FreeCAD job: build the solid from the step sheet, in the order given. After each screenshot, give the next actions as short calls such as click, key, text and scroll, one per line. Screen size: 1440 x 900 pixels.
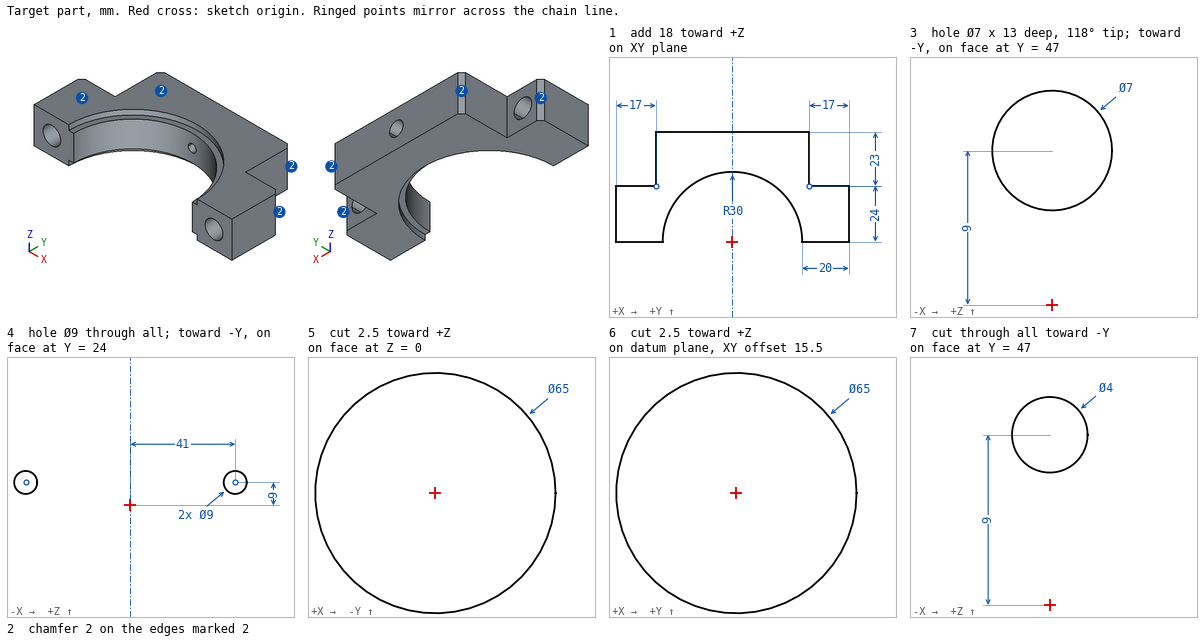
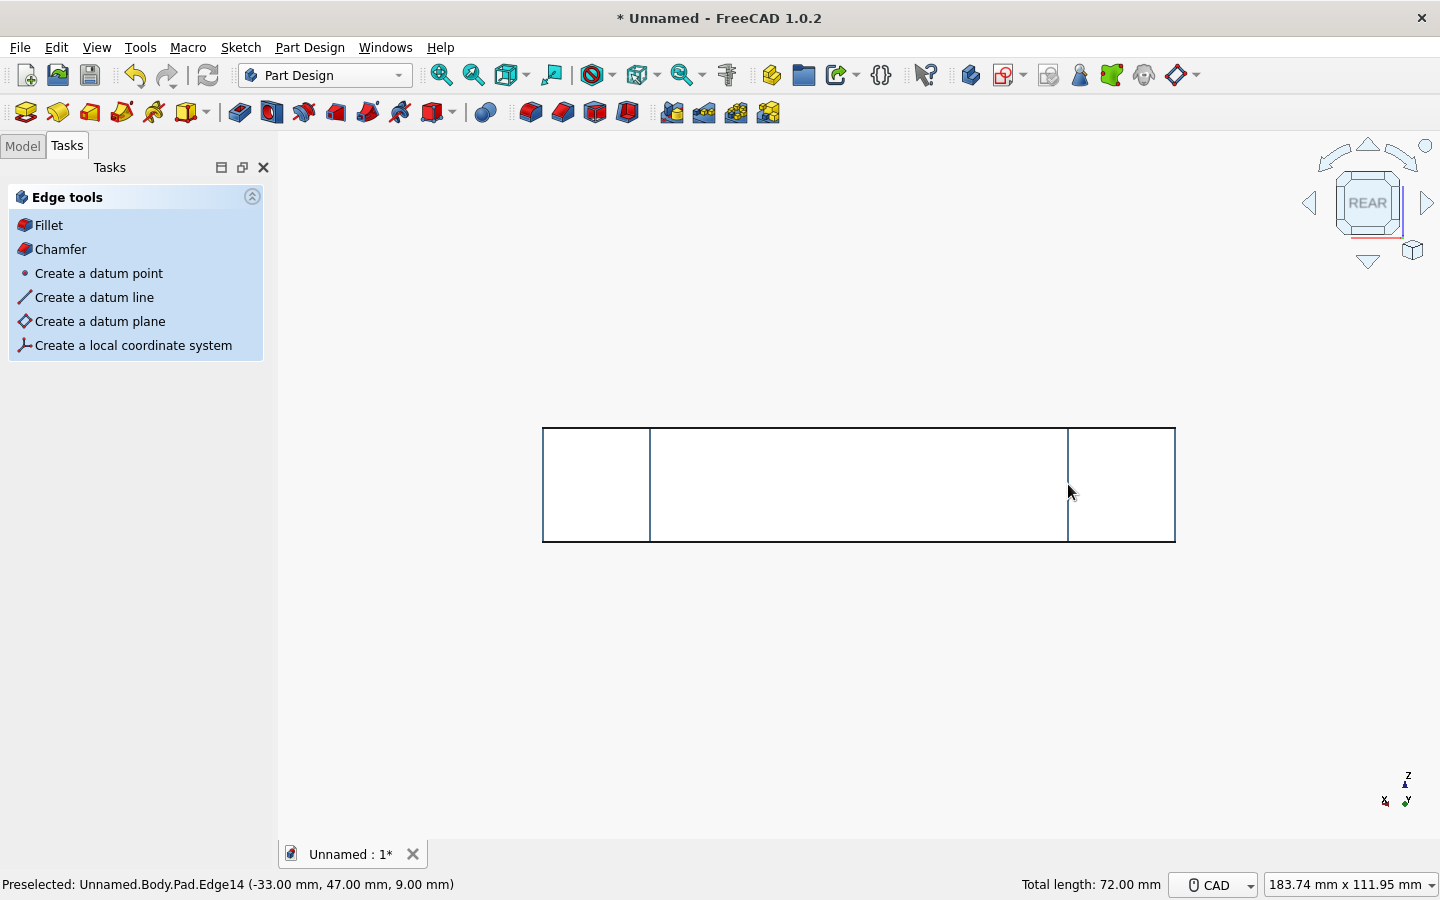
click(564, 112)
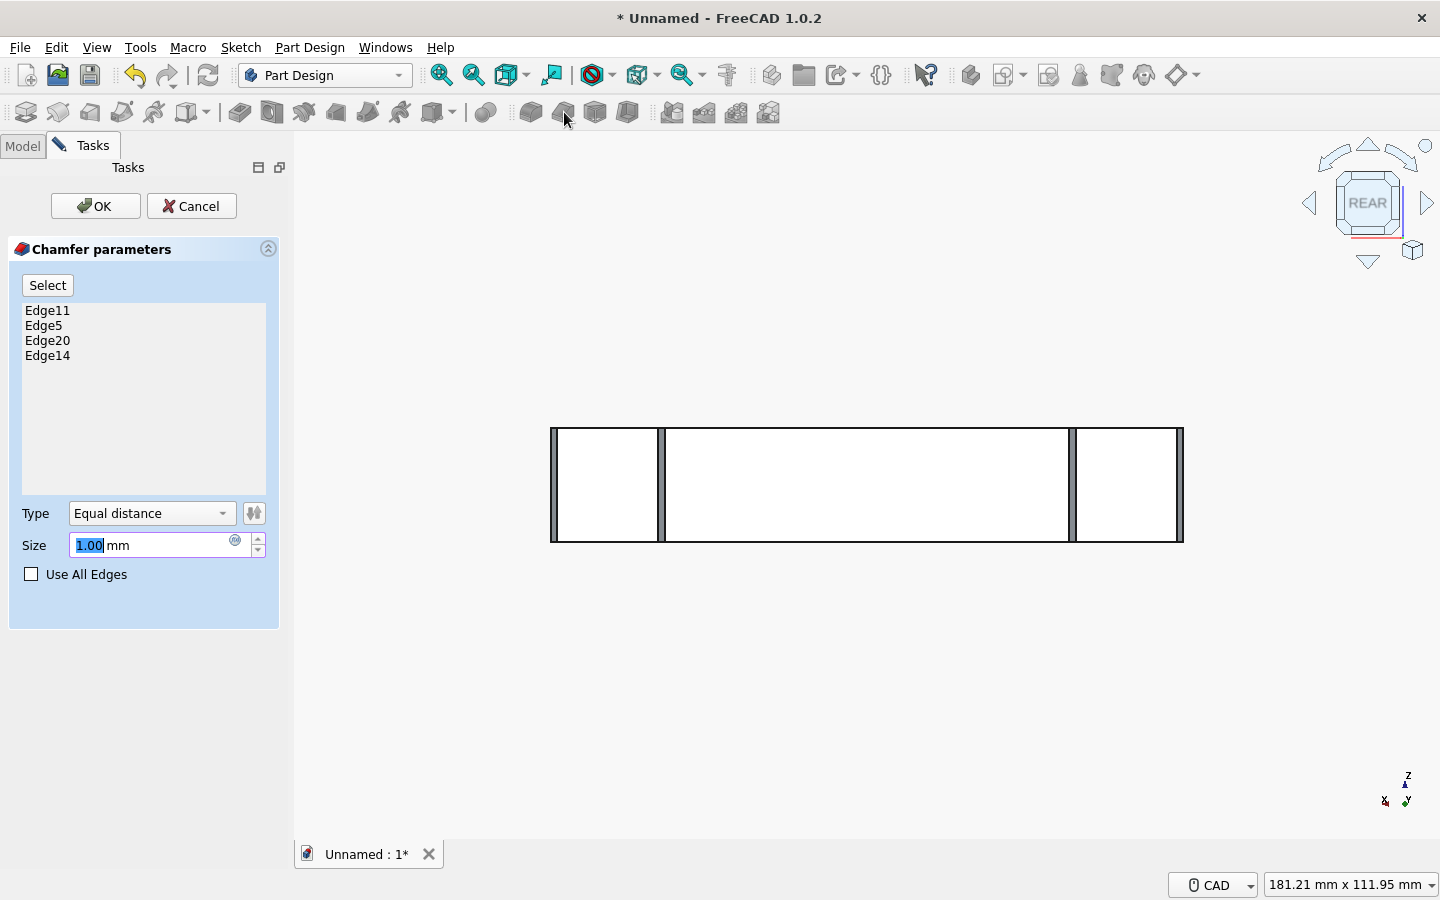
text(2)
key(Tab)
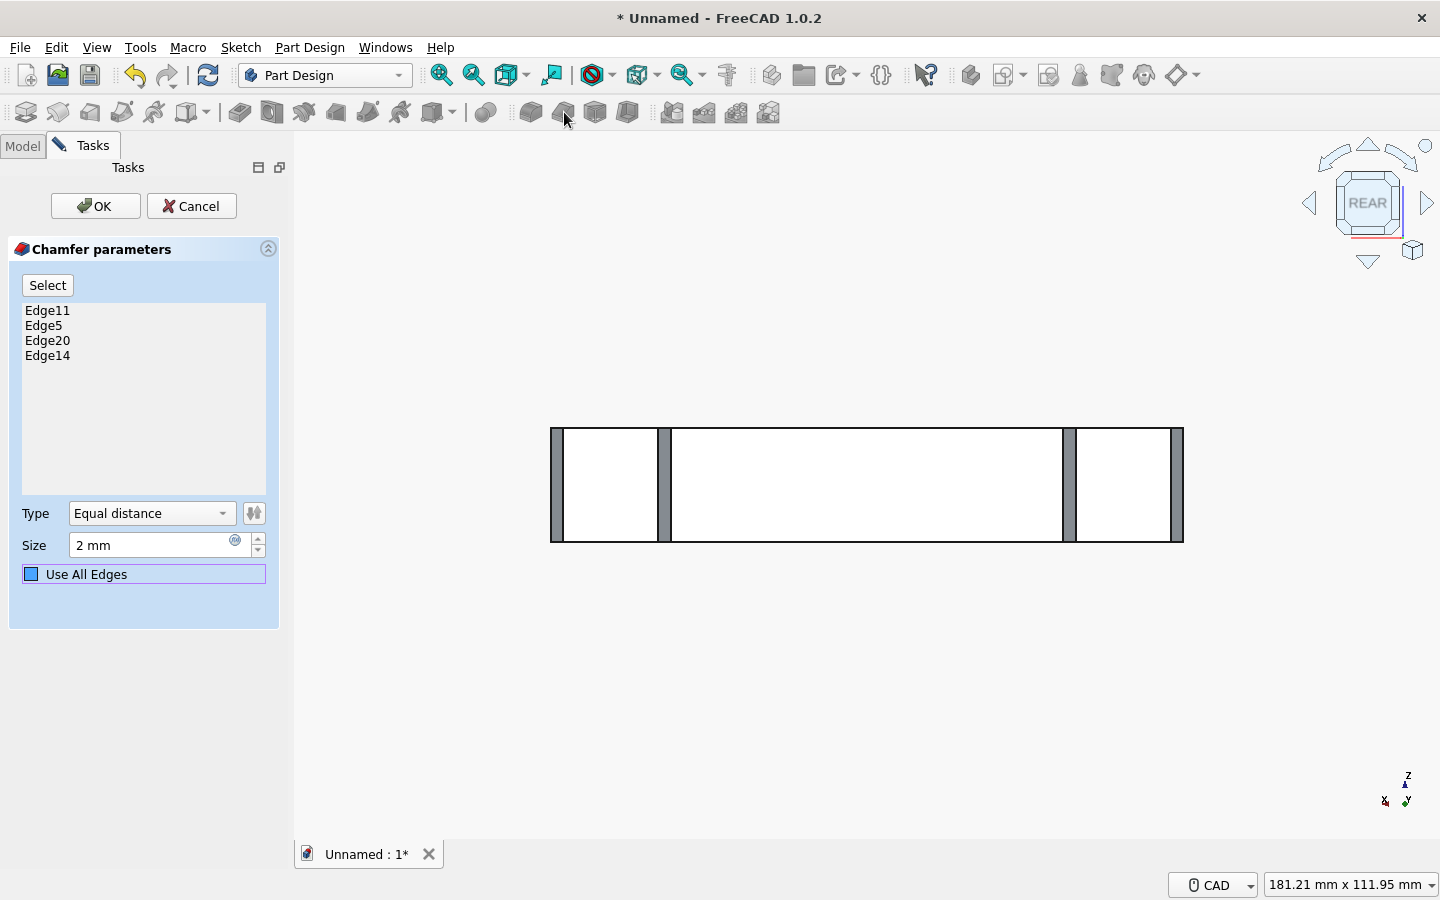
click(96, 206)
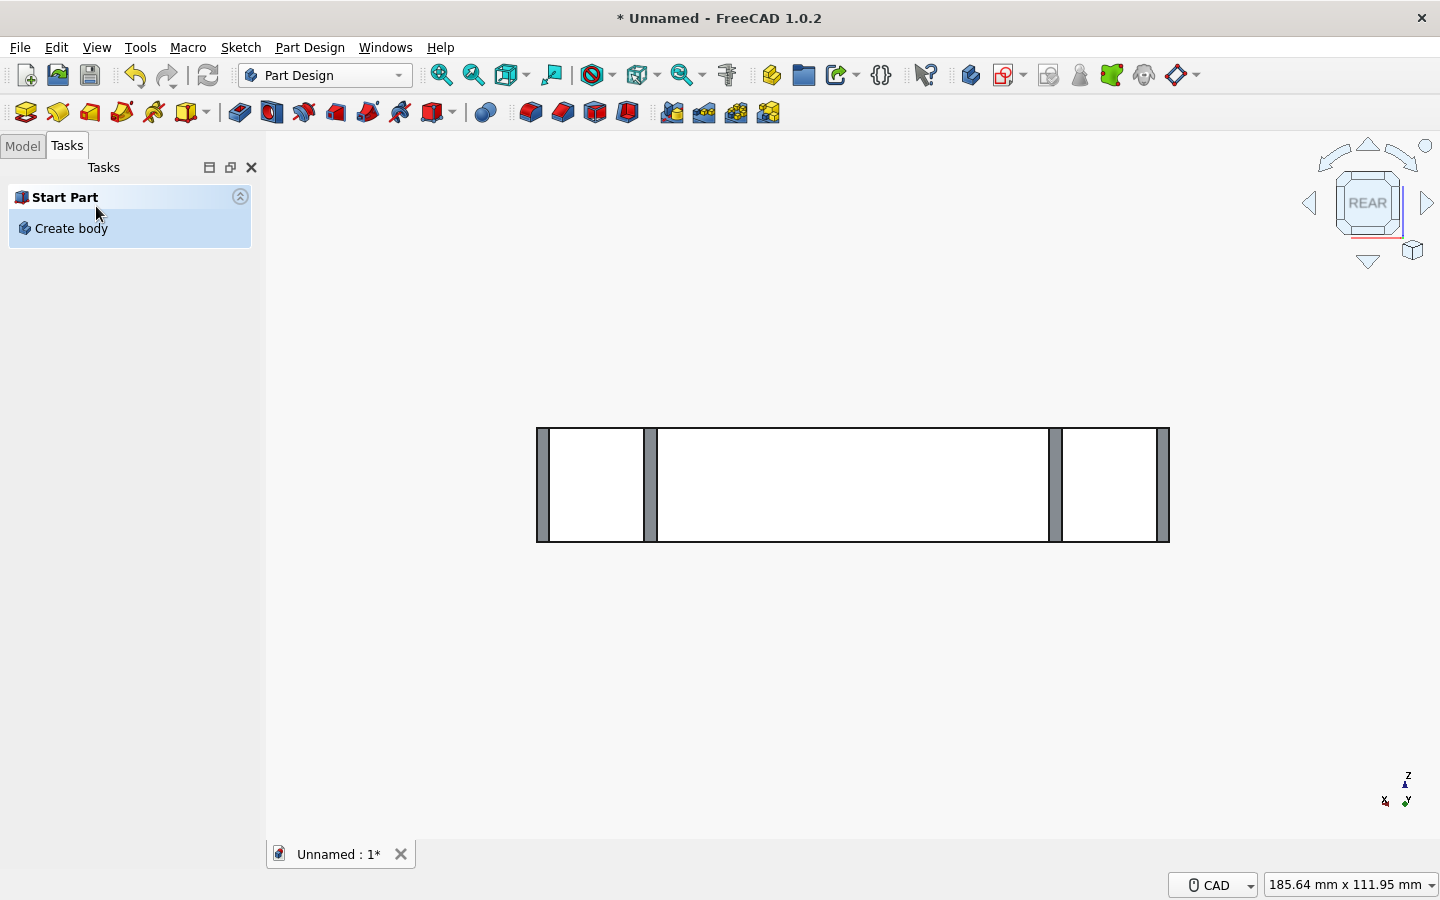
click(741, 484)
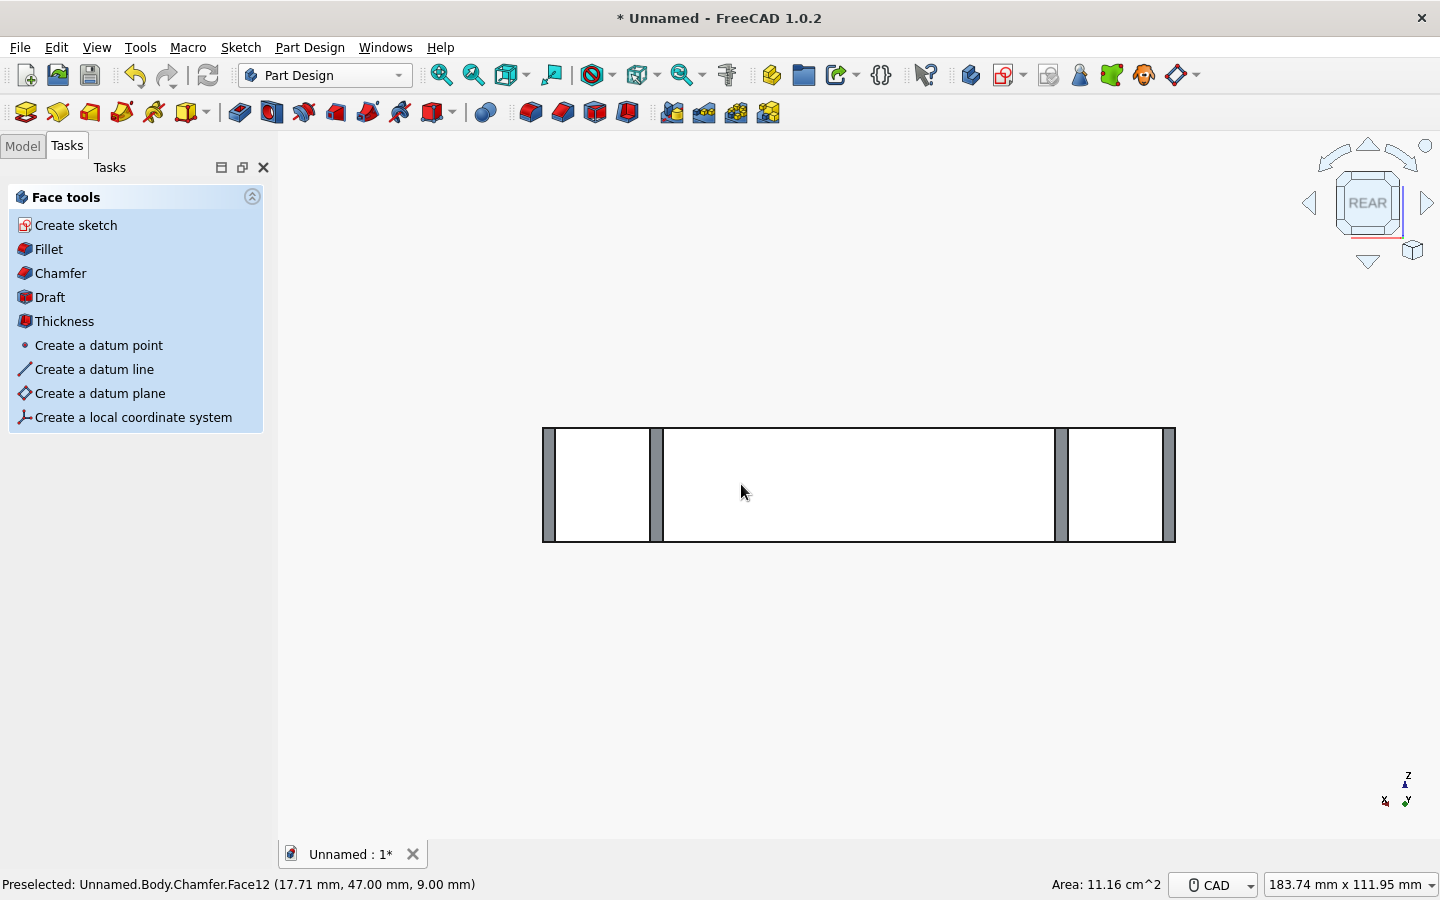
click(1004, 76)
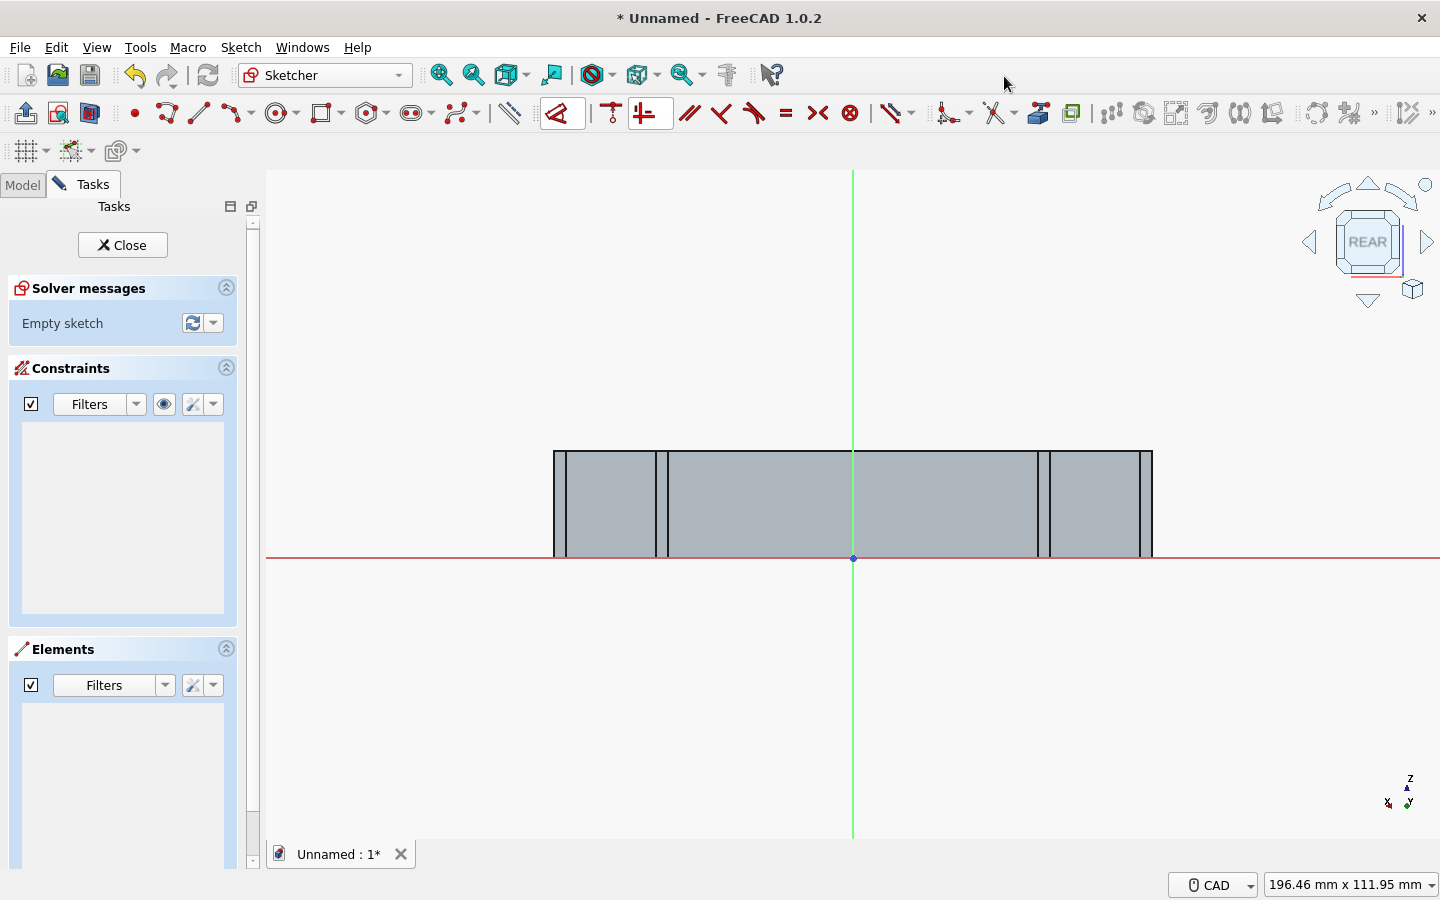
scroll(867, 524, up, 9)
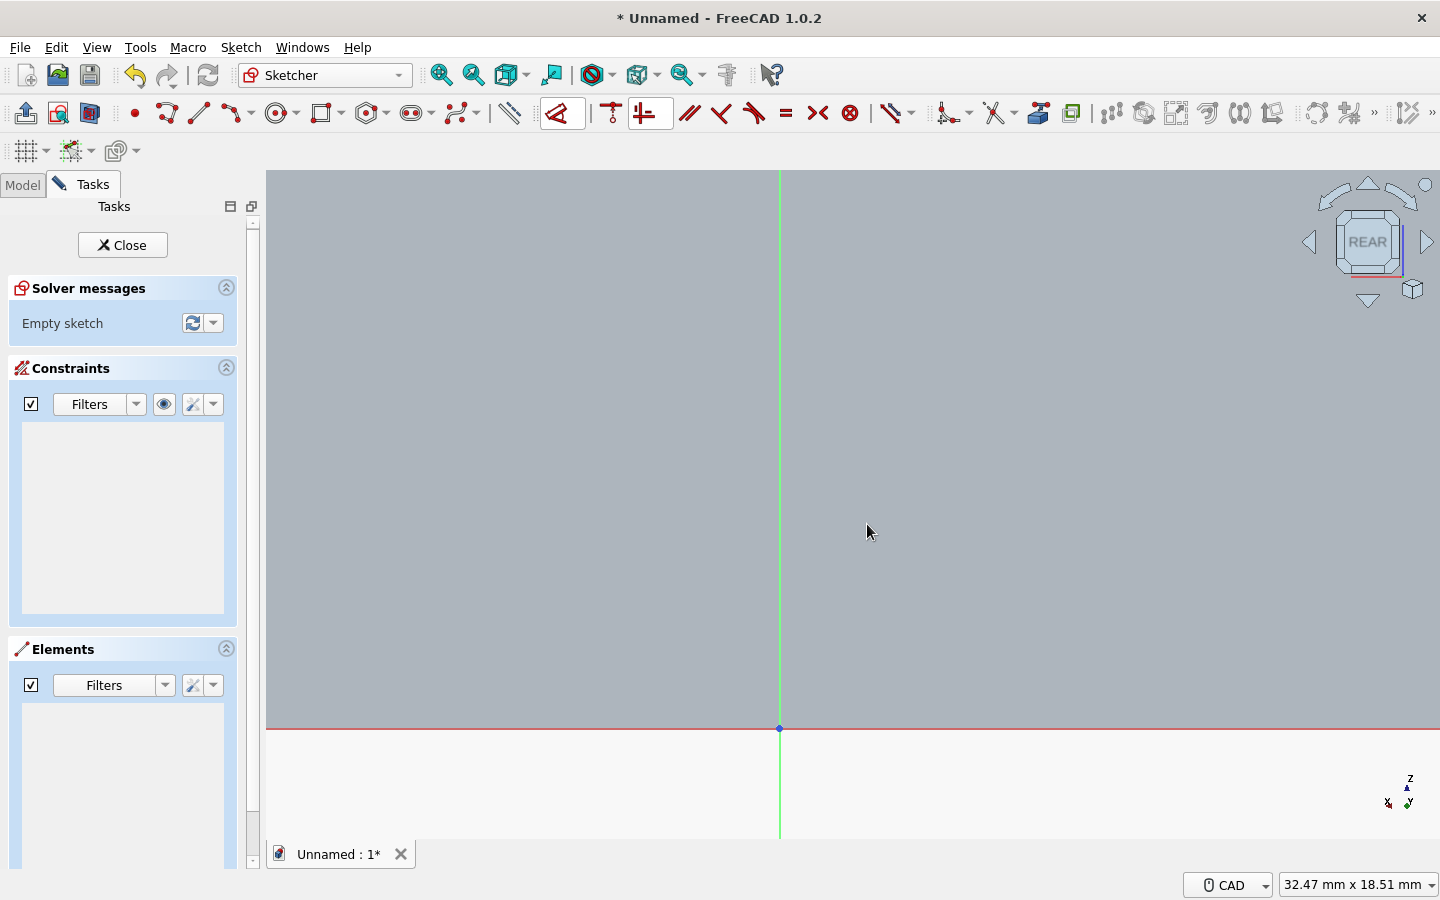
key(g)
key(c)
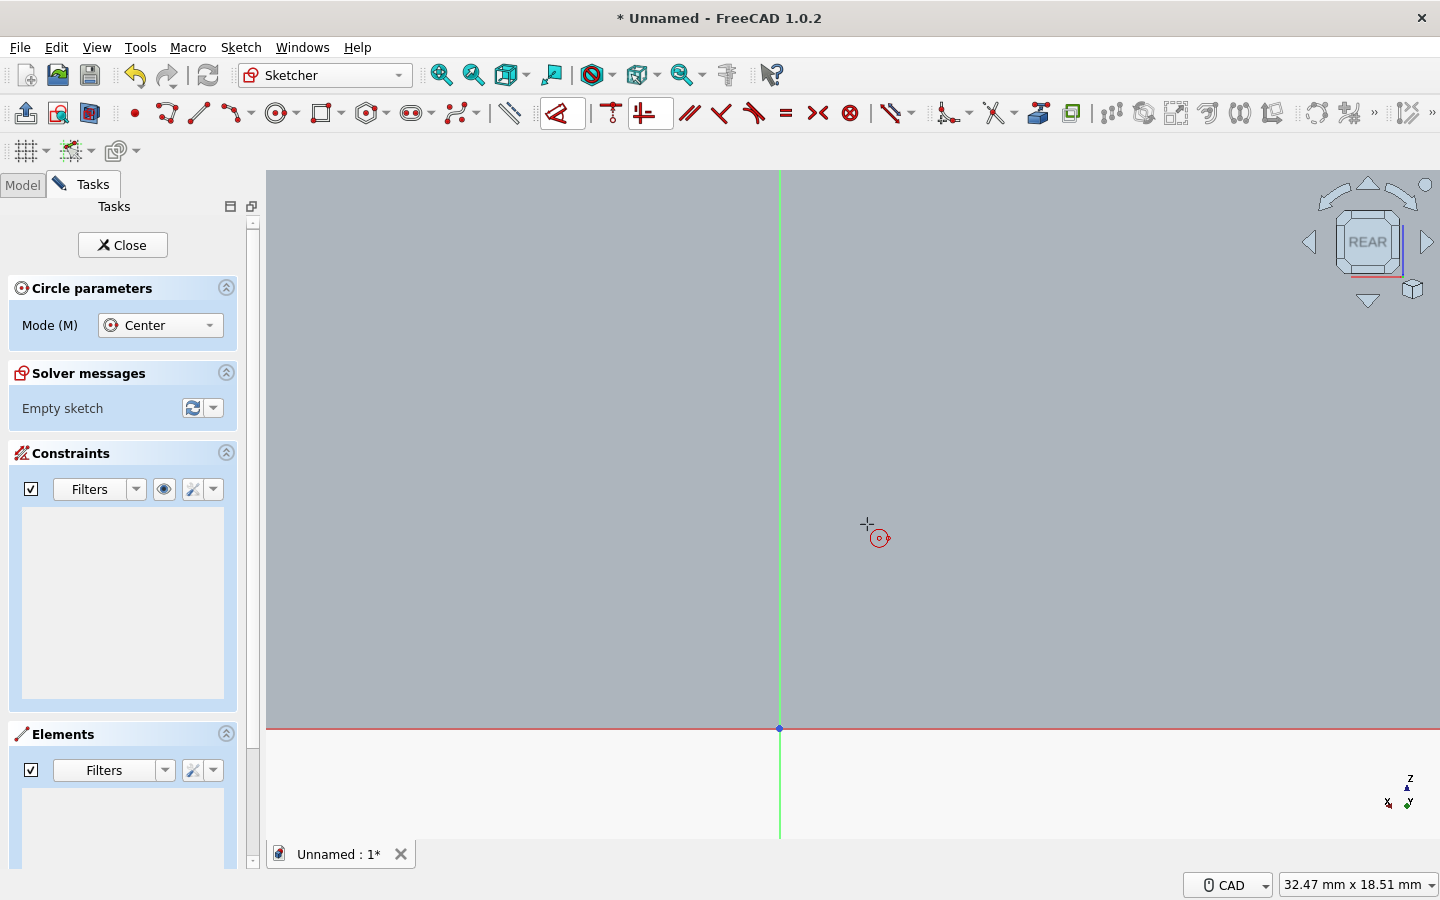
click(780, 403)
click(869, 314)
key(Escape)